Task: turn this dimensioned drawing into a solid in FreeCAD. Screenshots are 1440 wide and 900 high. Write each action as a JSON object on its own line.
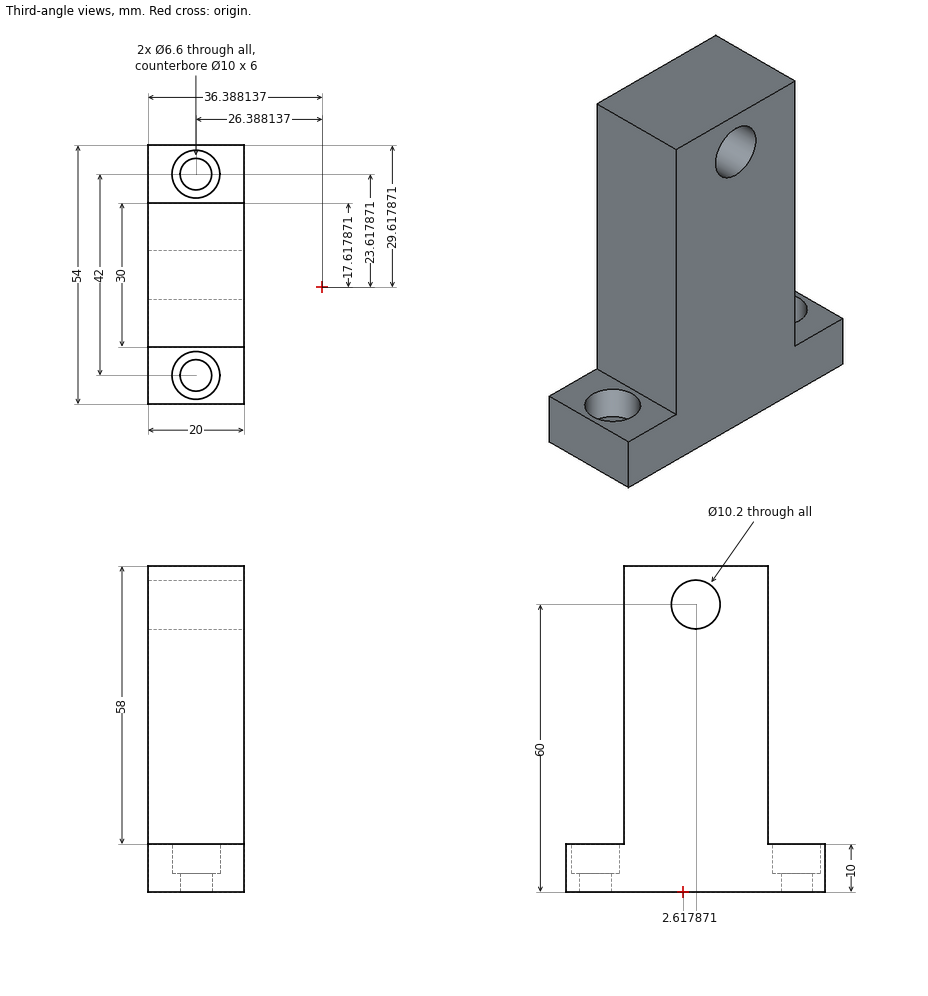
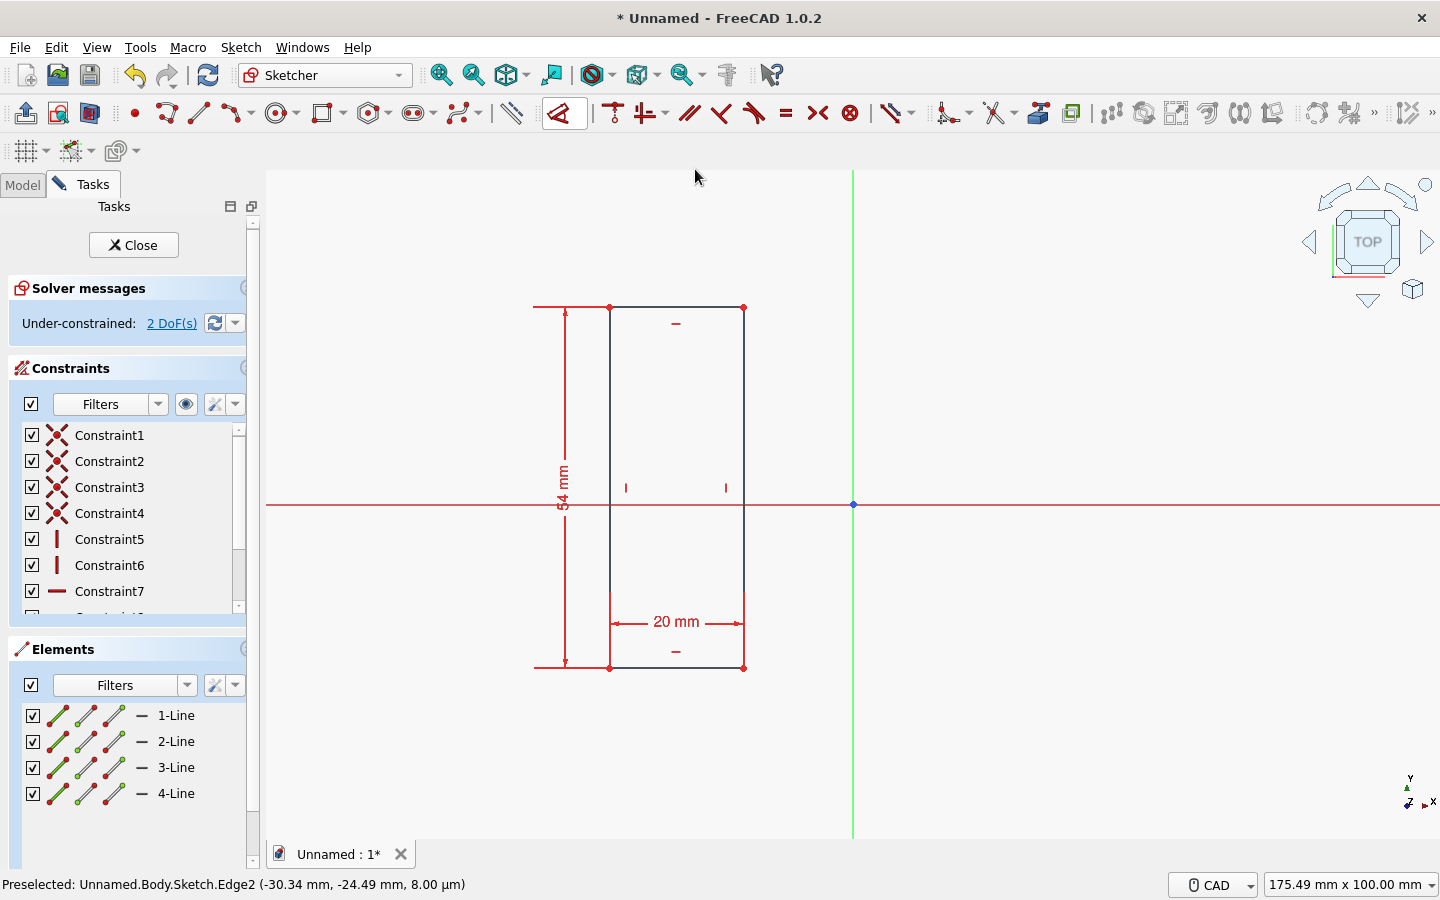
{"action": "left_click", "coordinate": [610, 307]}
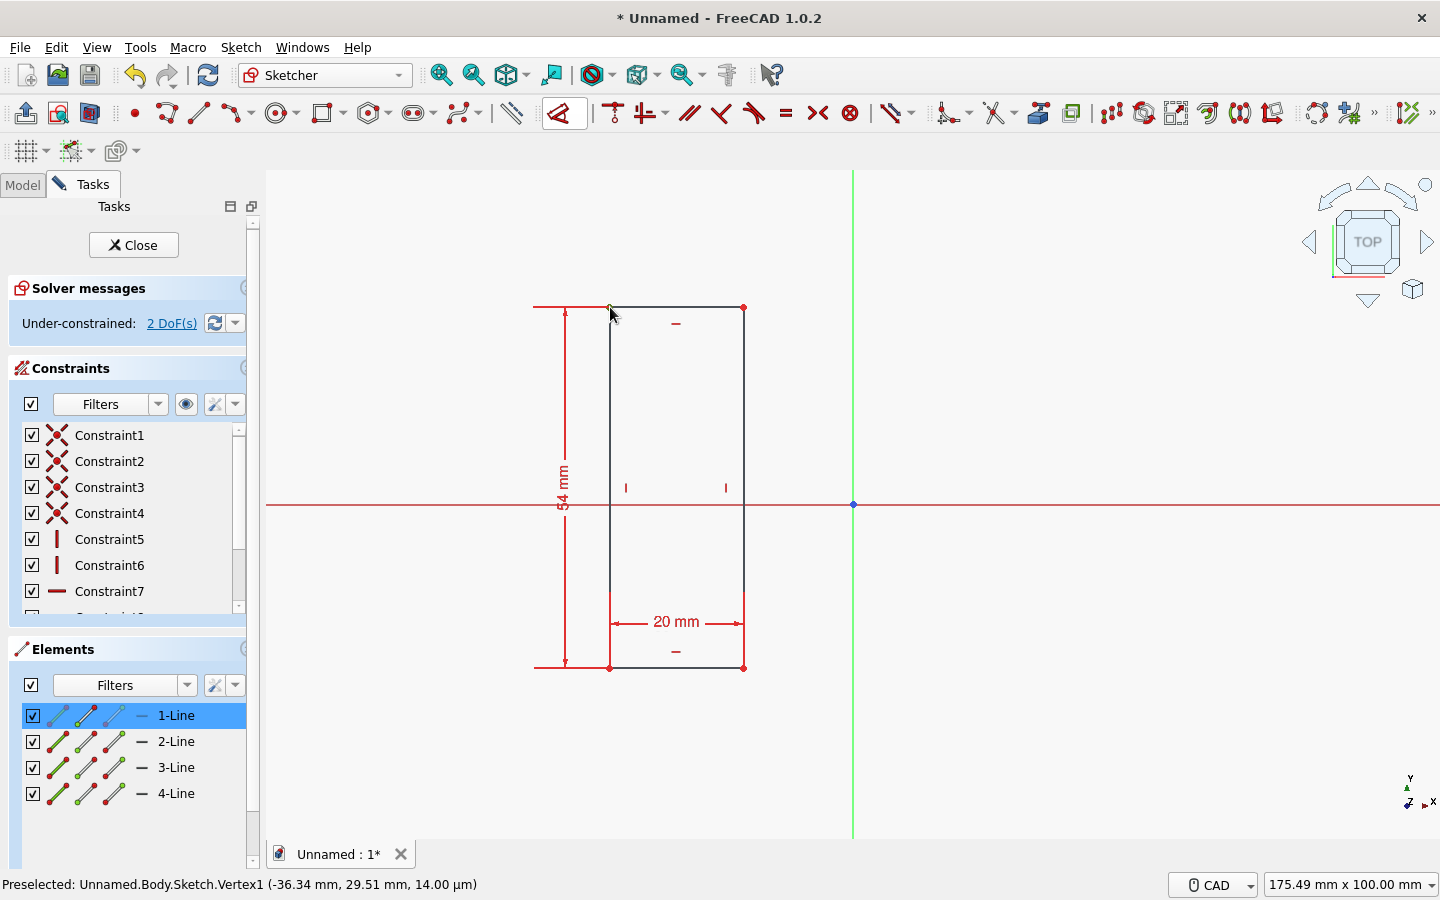
{"action": "key", "text": "l"}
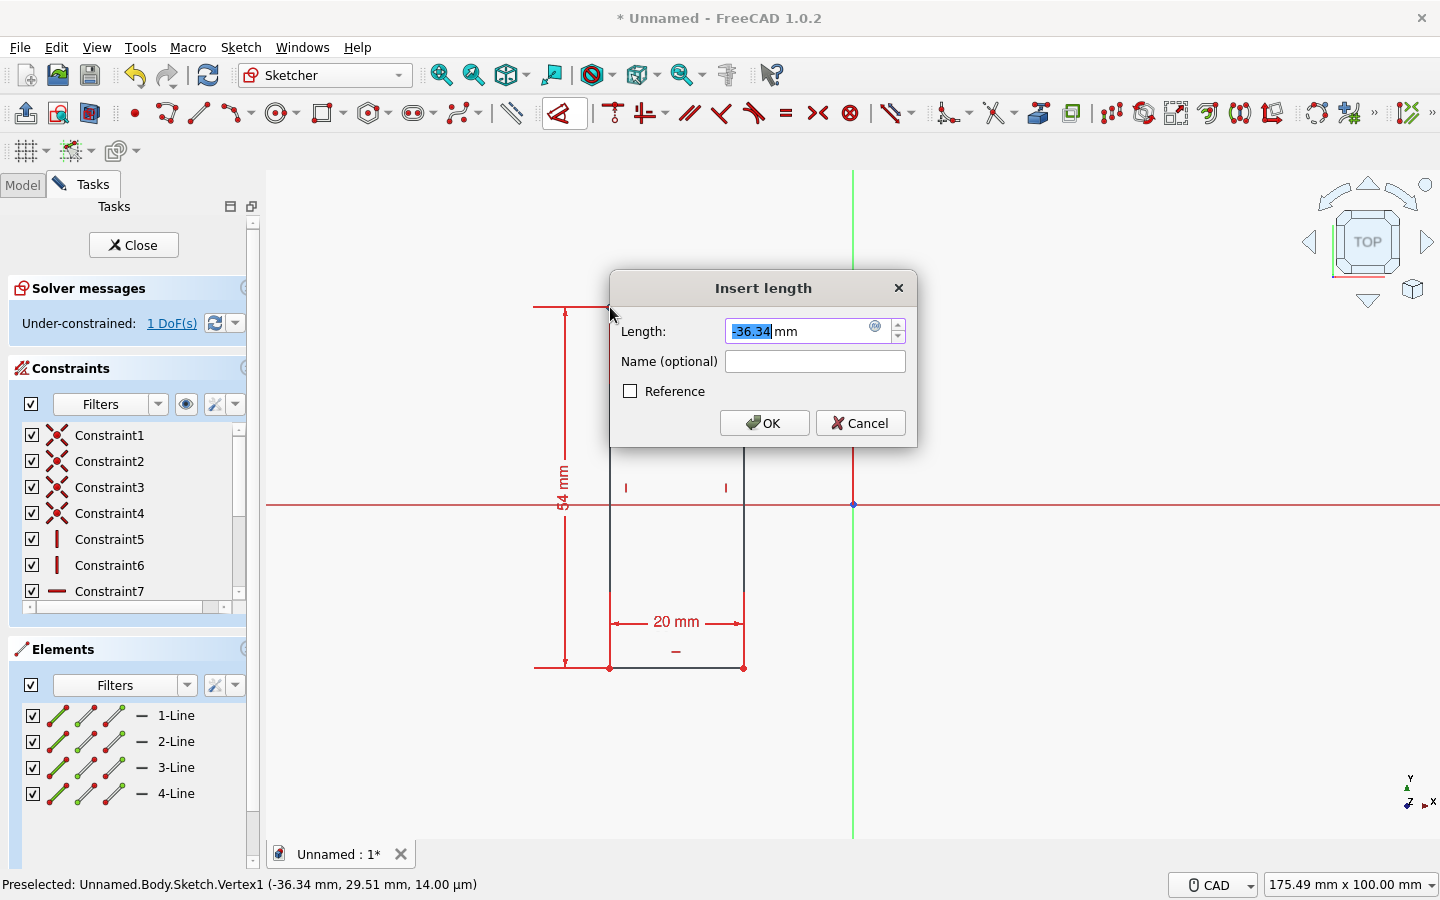
{"action": "type", "text": "-36.388137"}
{"action": "key", "text": "Return"}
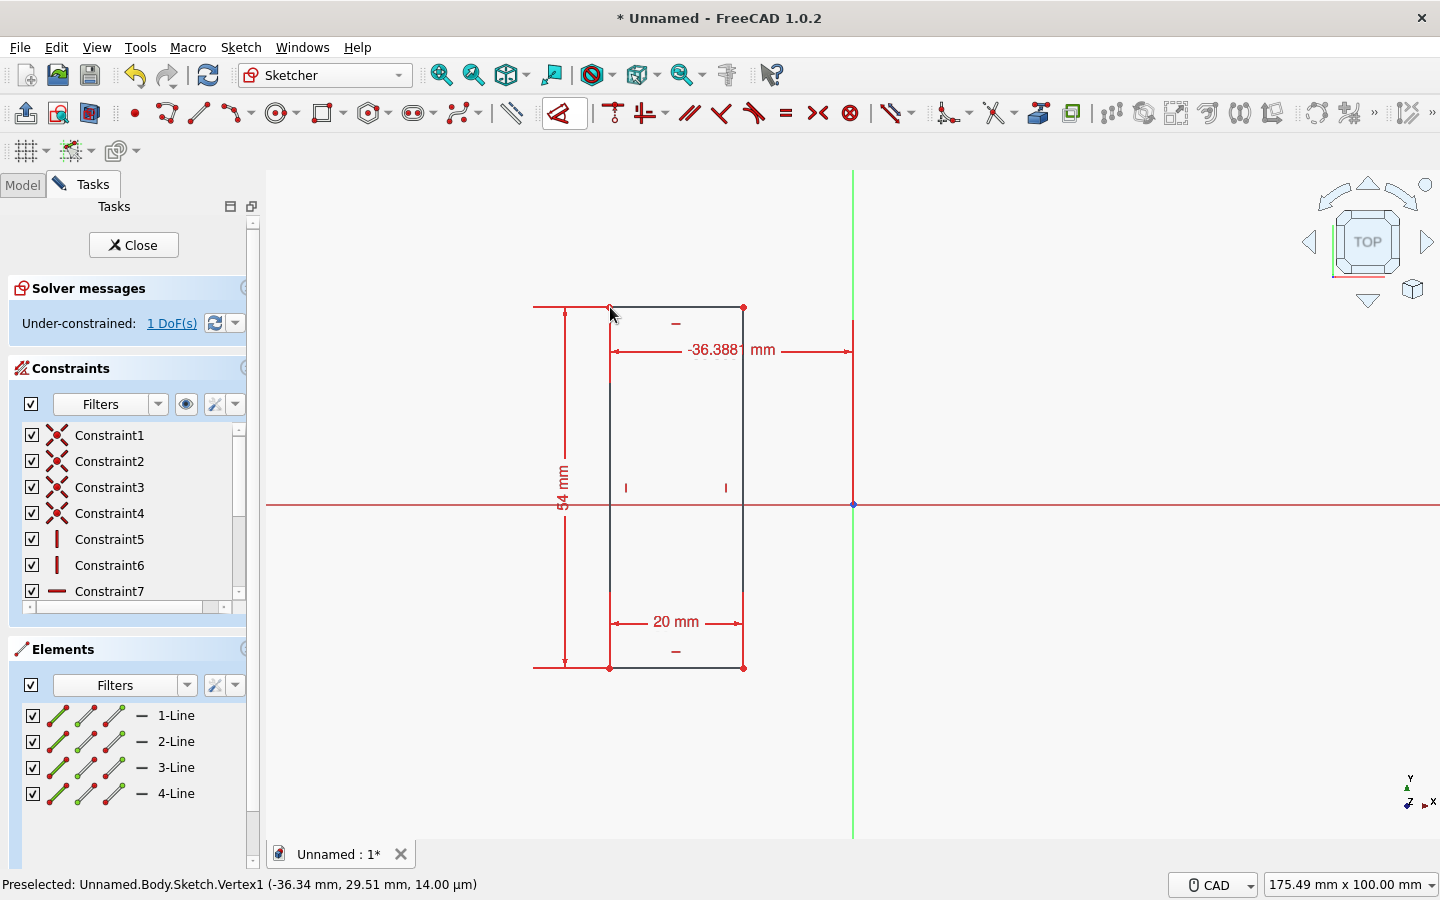
{"action": "left_click", "coordinate": [610, 307]}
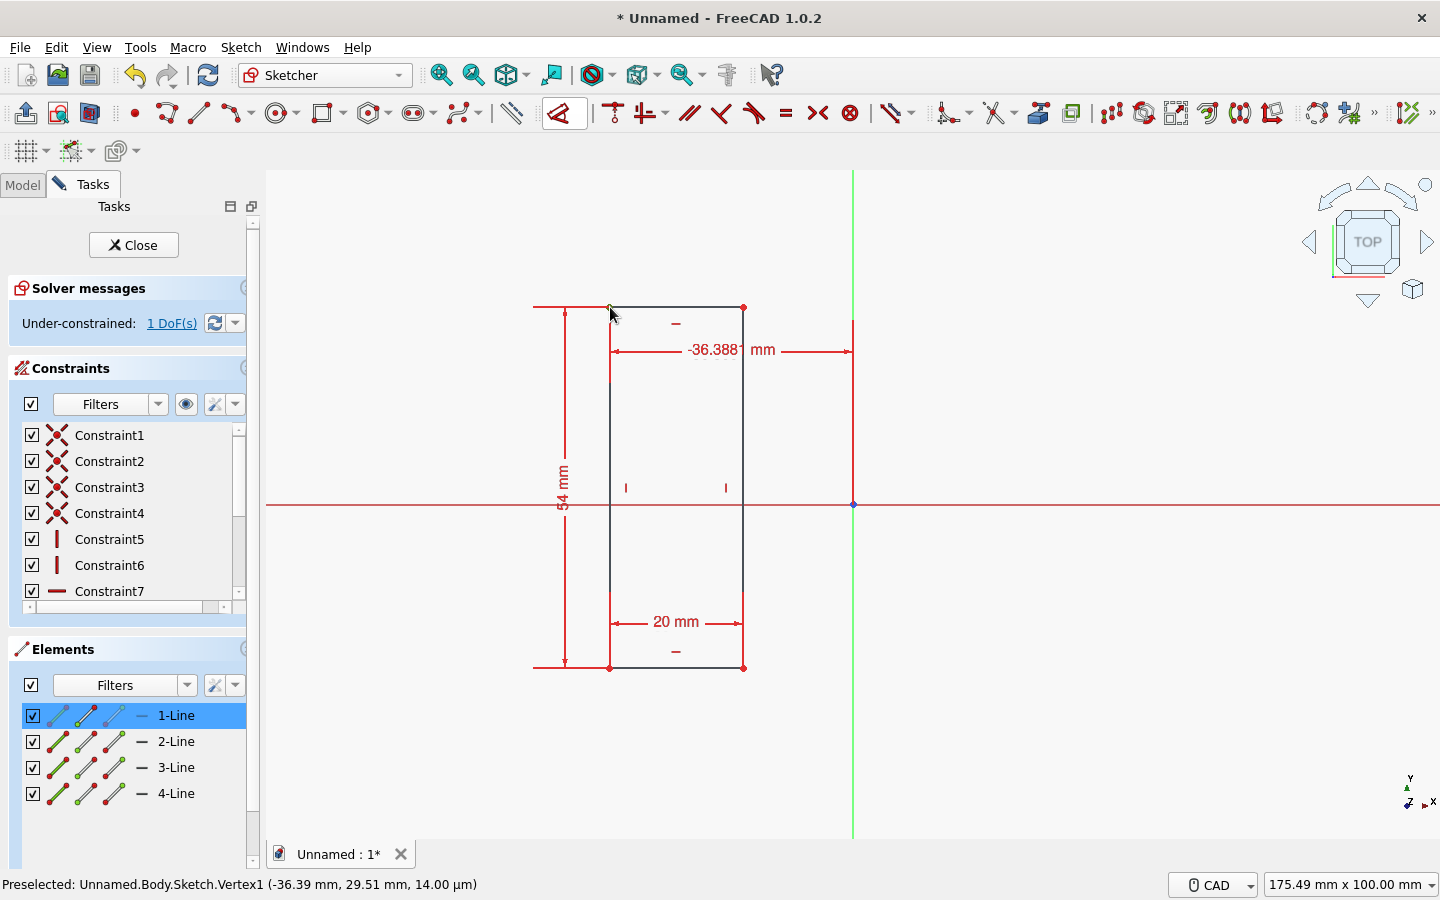
{"action": "key", "text": "i"}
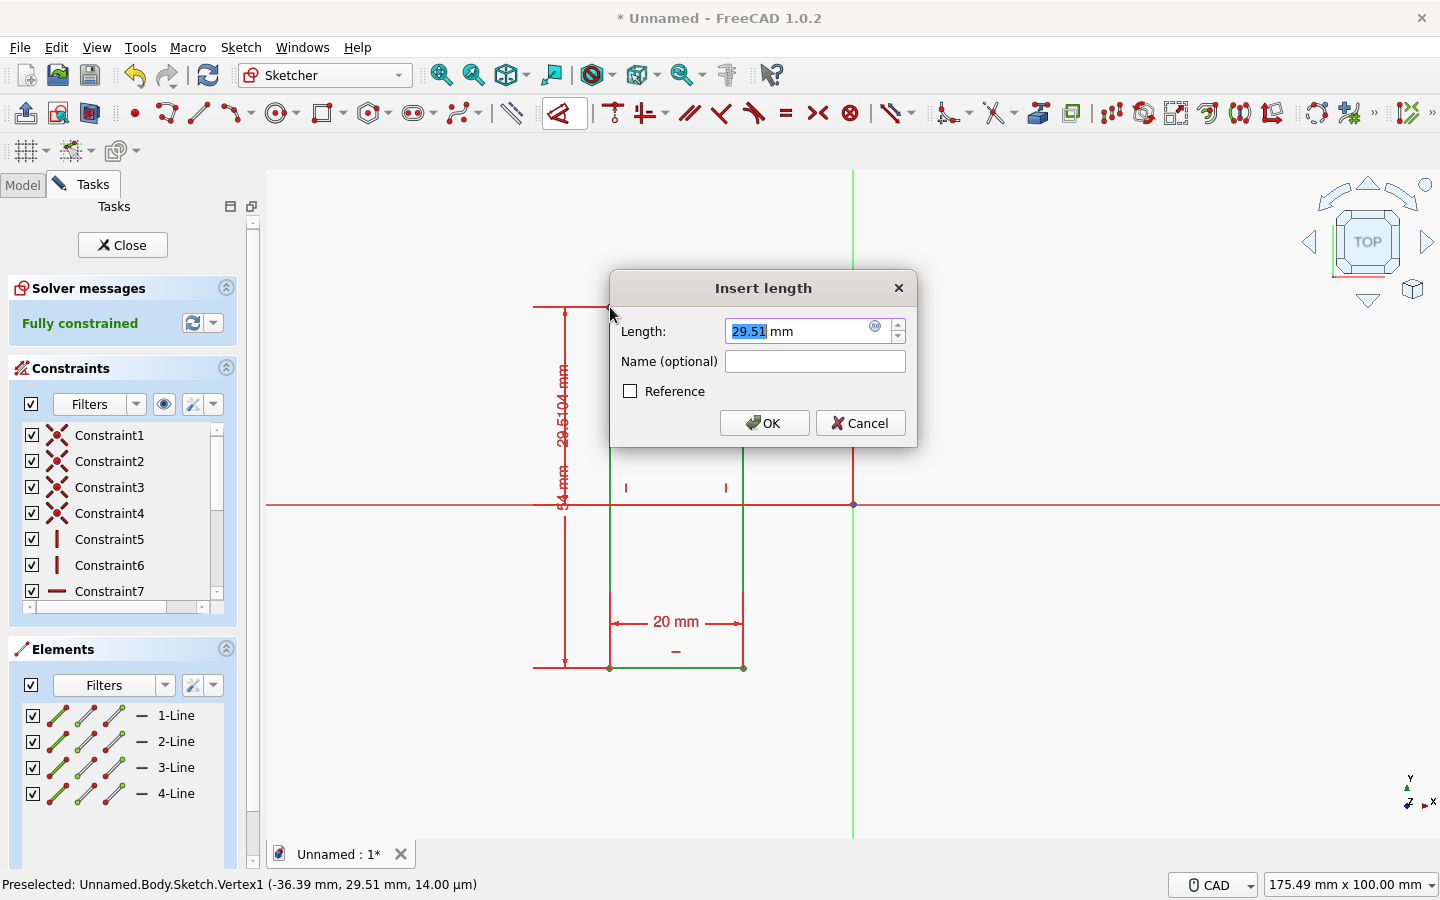
{"action": "type", "text": "29.617871"}
{"action": "key", "text": "Return"}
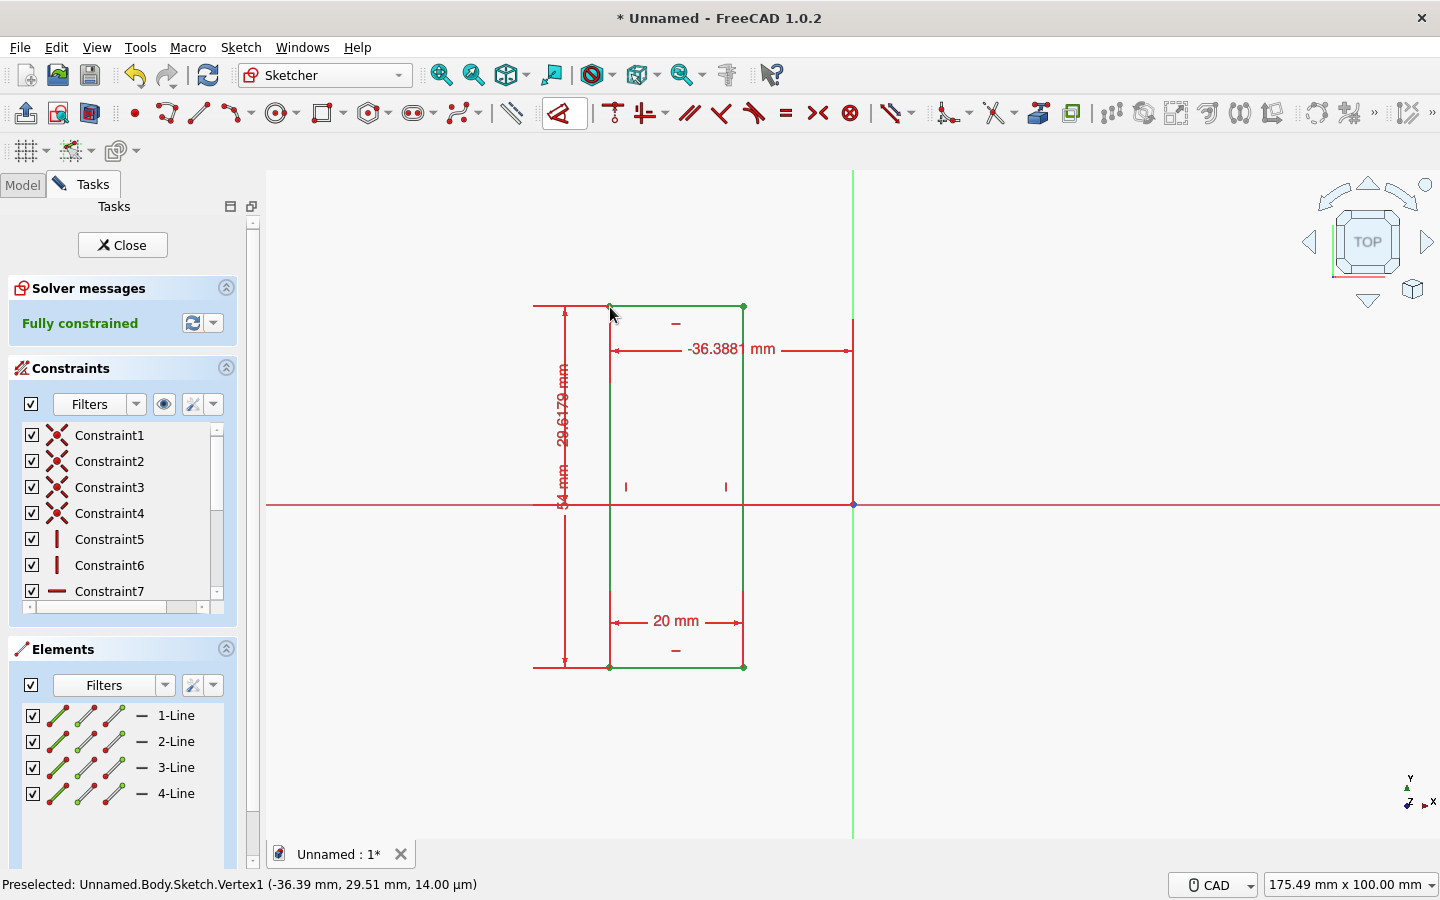
{"action": "left_click", "coordinate": [123, 245]}